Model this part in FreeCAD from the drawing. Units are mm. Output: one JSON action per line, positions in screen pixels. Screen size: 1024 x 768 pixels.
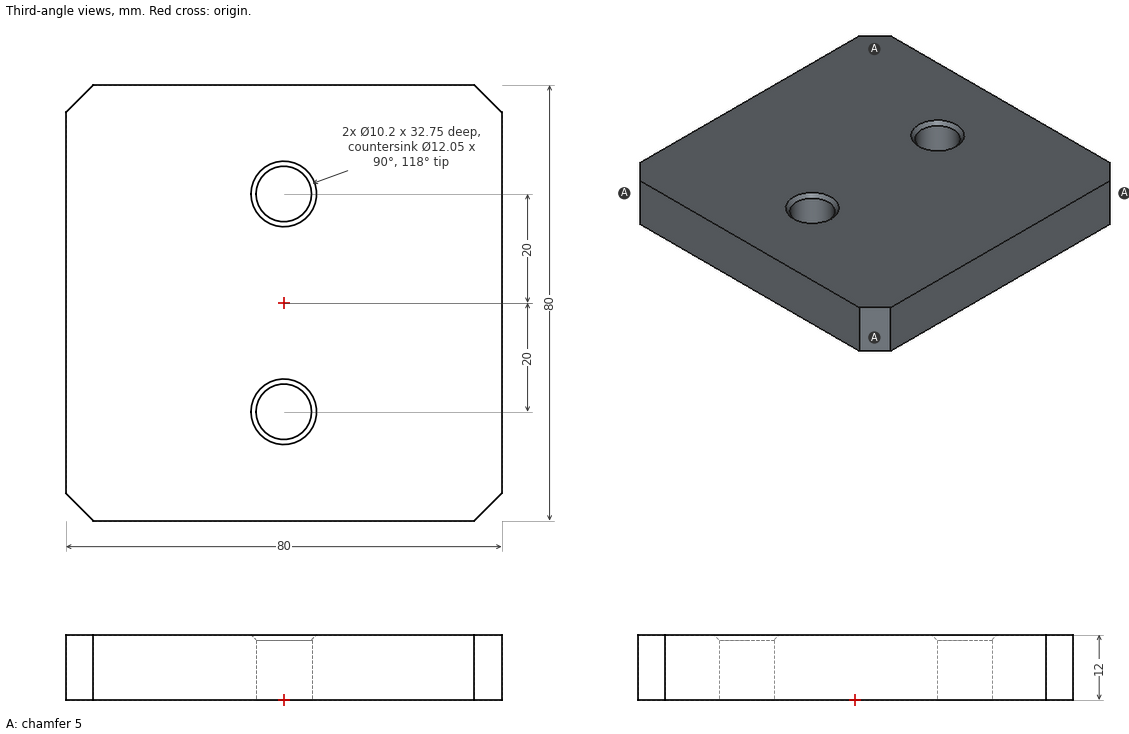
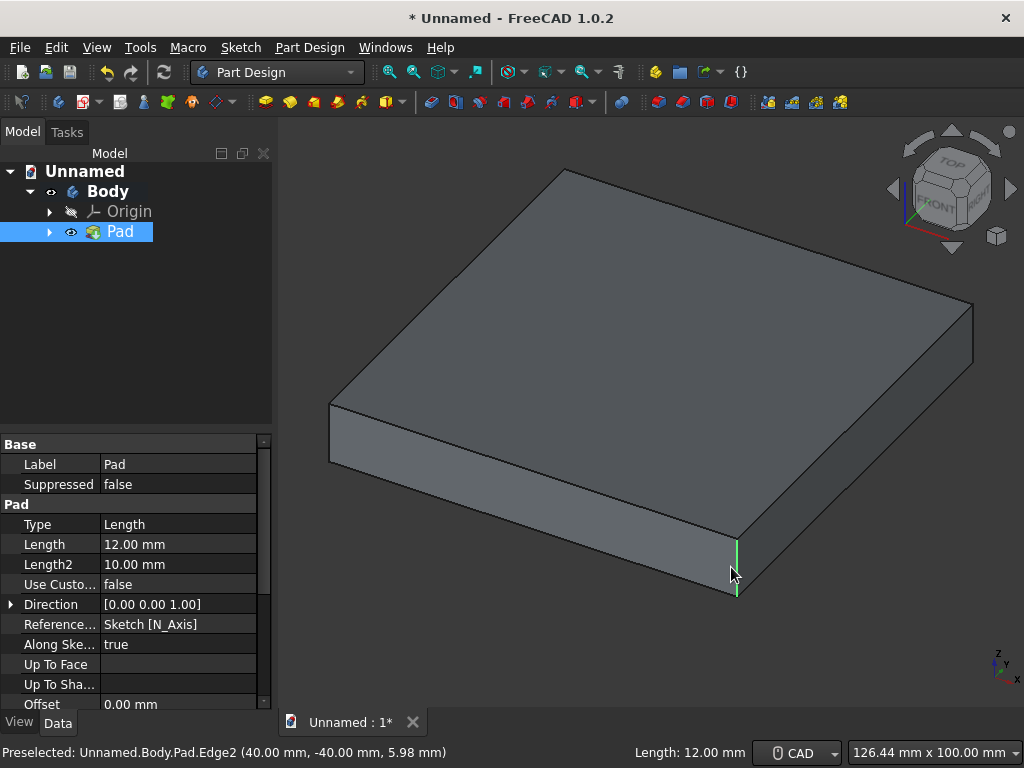
{"action": "key", "text": "0"}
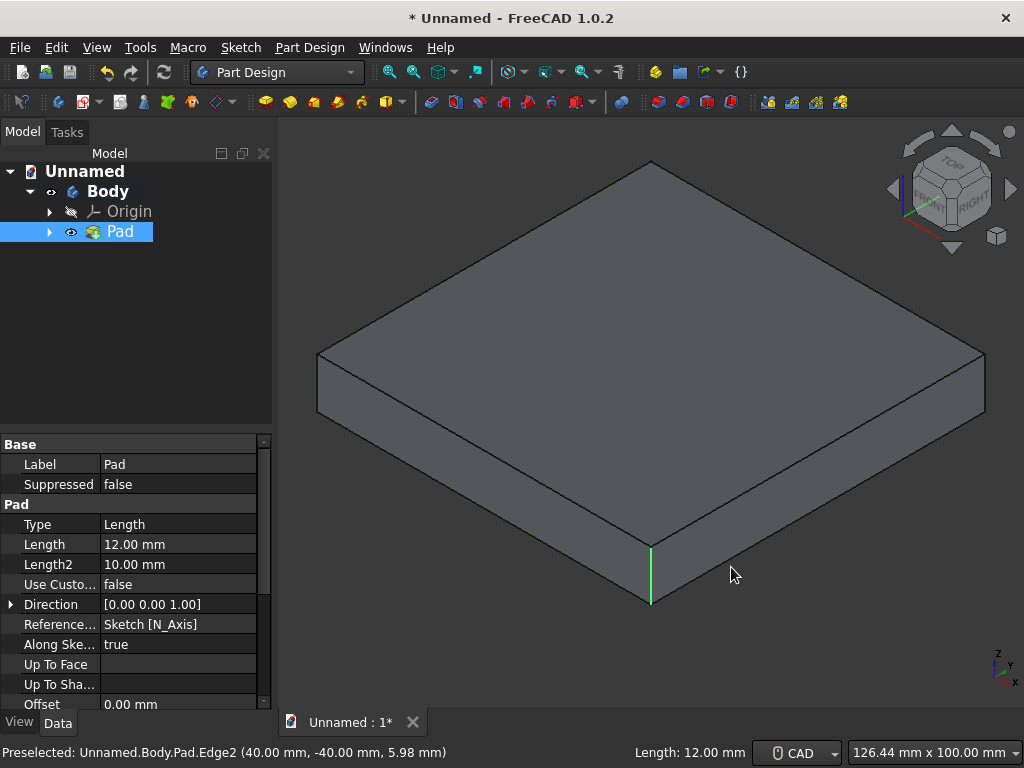
{"action": "key", "text": "2"}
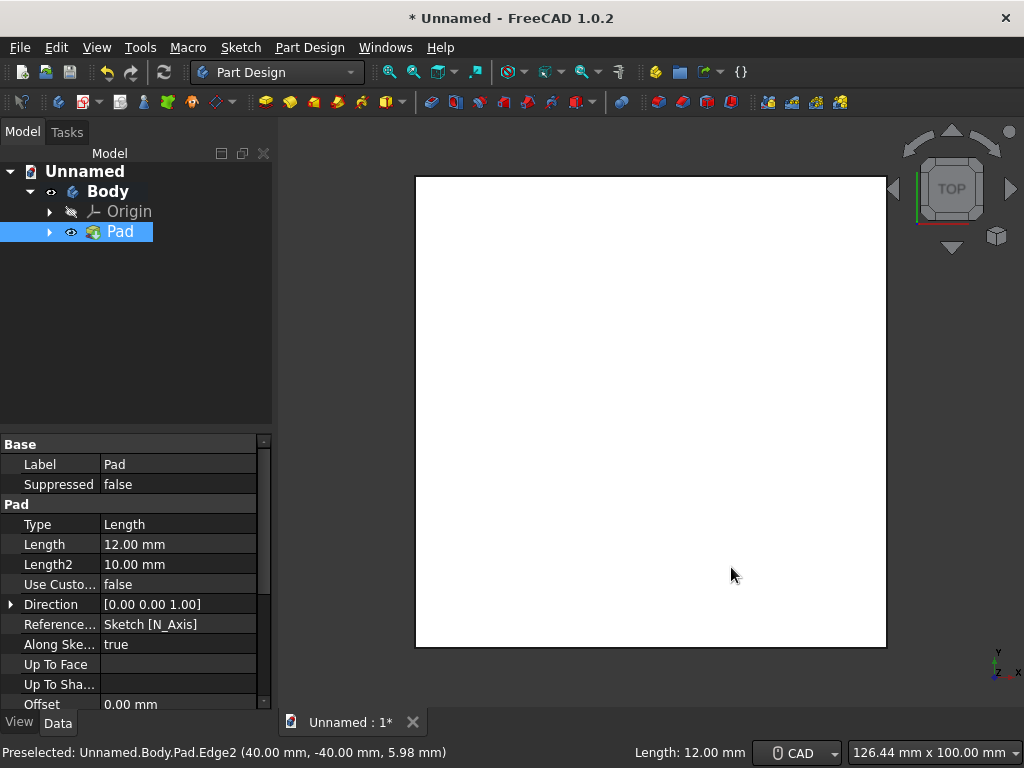
{"action": "key", "text": "1"}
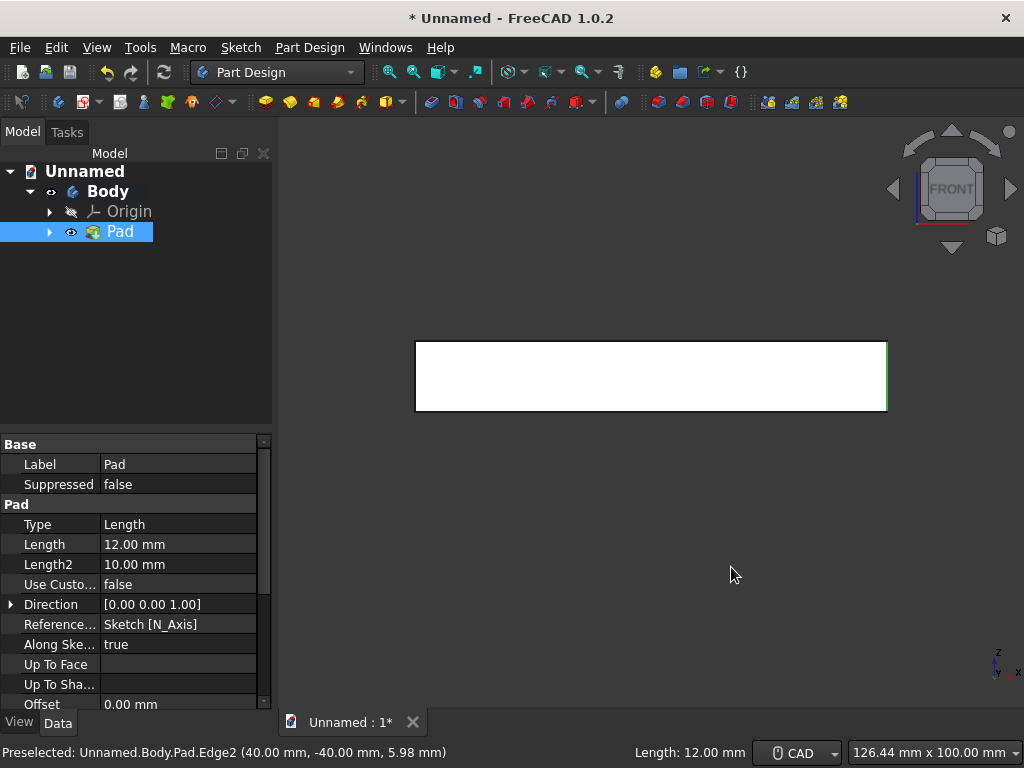
{"action": "left_click", "coordinate": [415, 376], "text": "ctrl"}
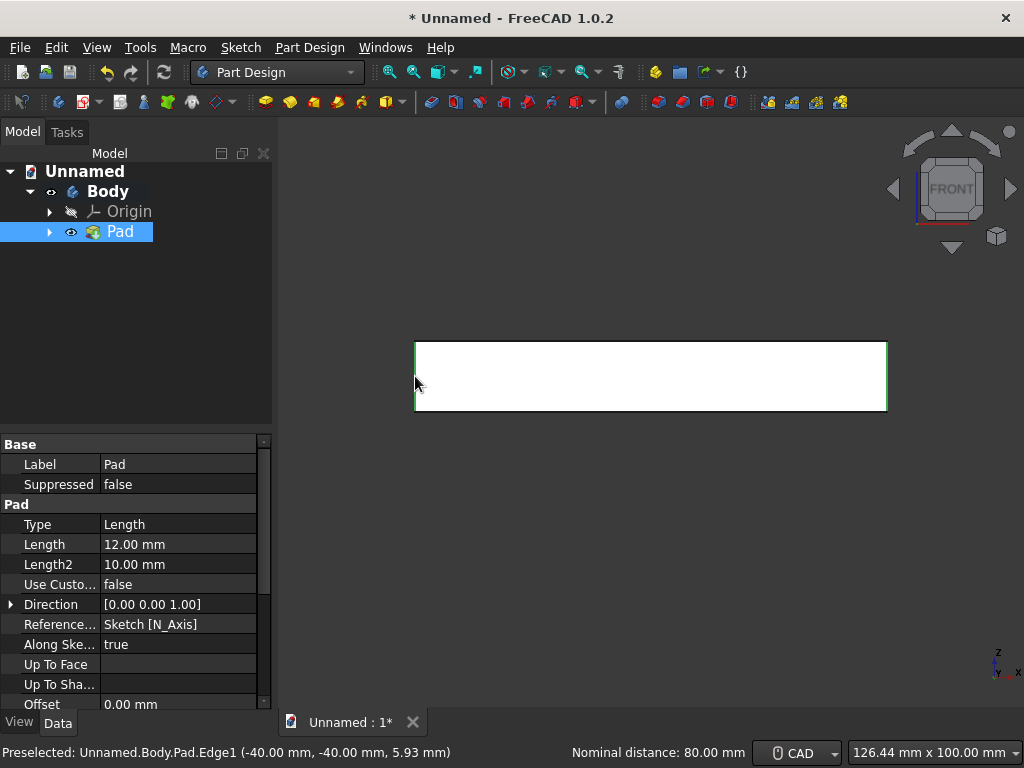
{"action": "key", "text": "3"}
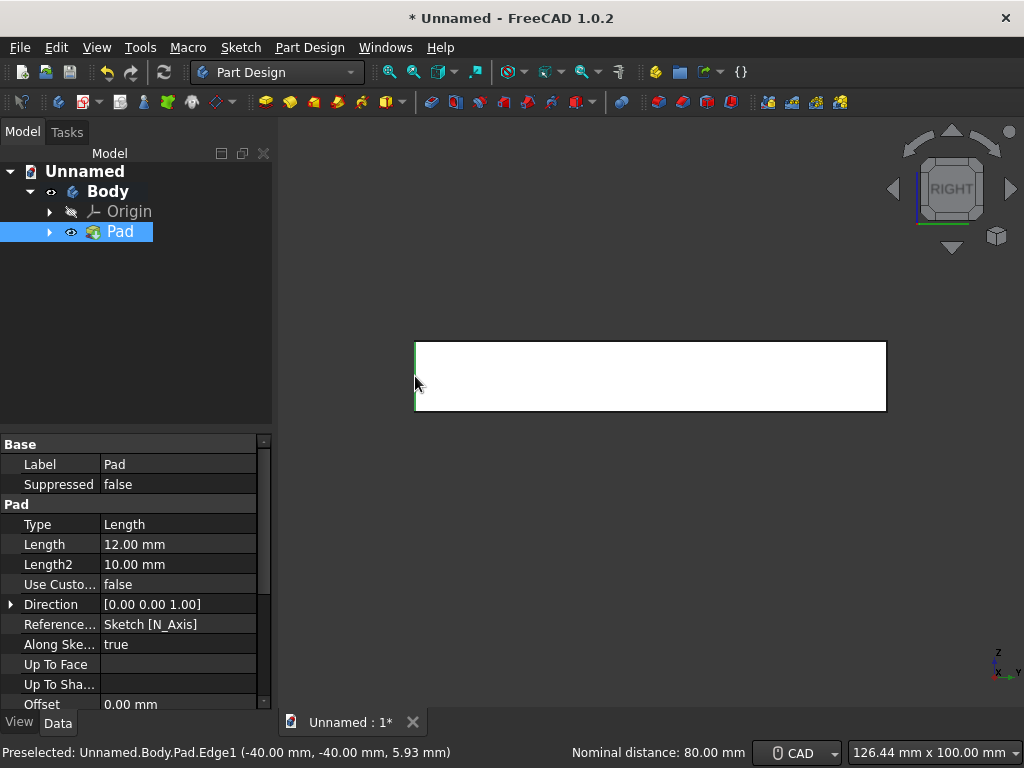
{"action": "left_click", "coordinate": [887, 376], "text": "ctrl"}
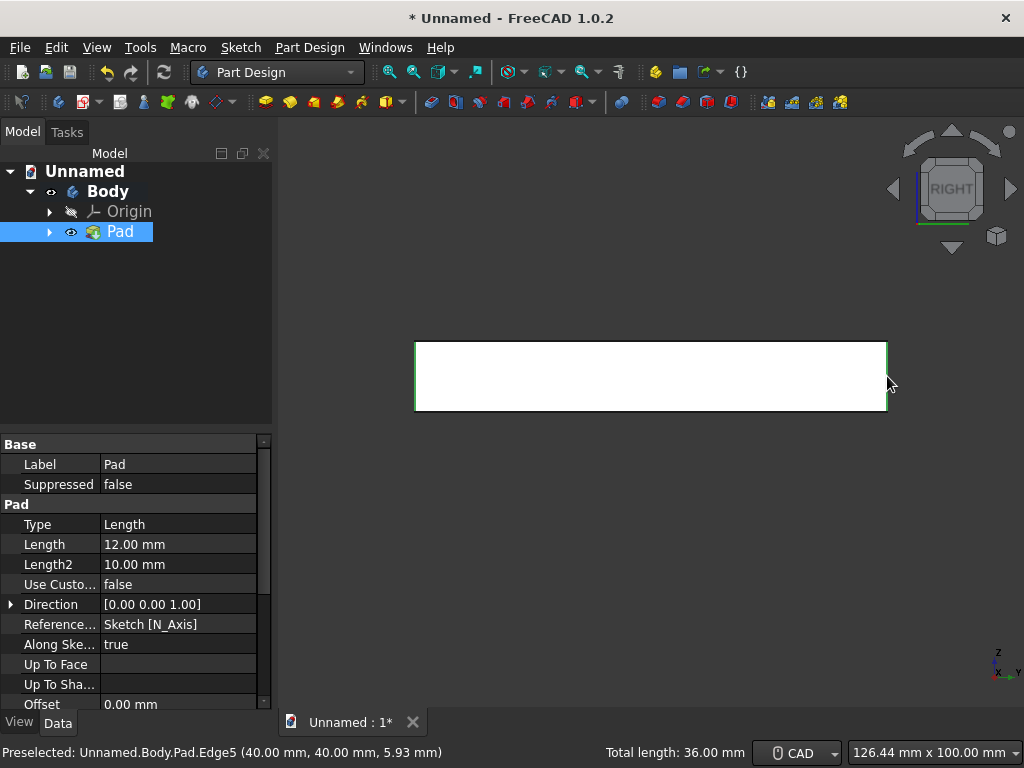
{"action": "key", "text": "5"}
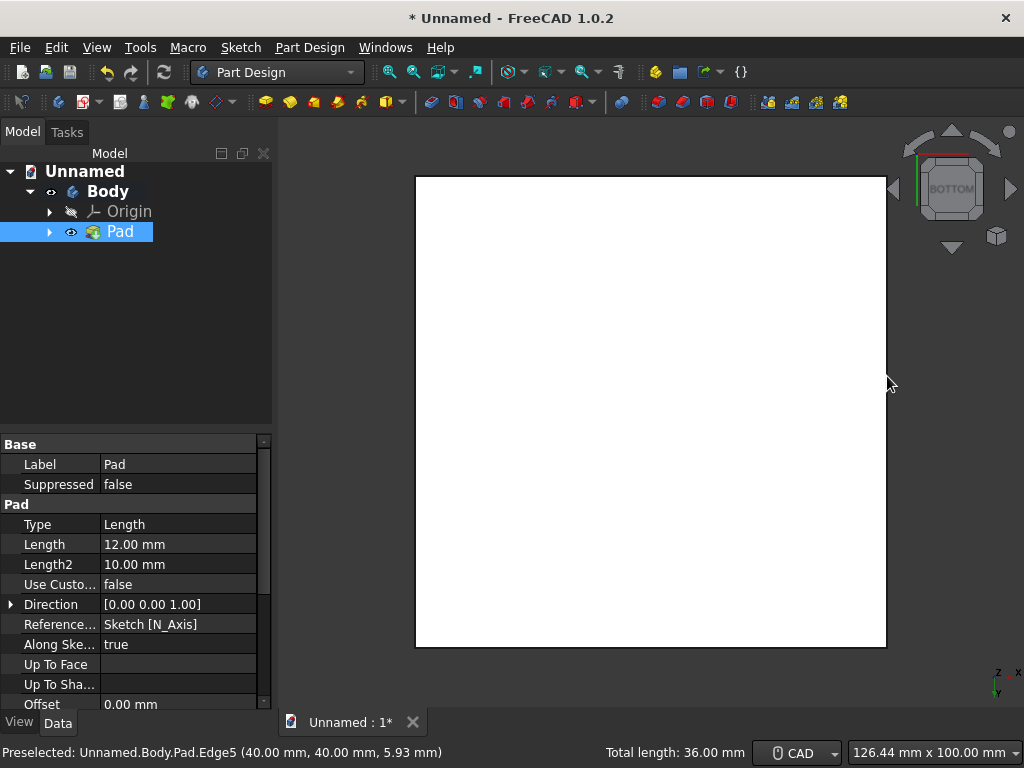
{"action": "key", "text": "4"}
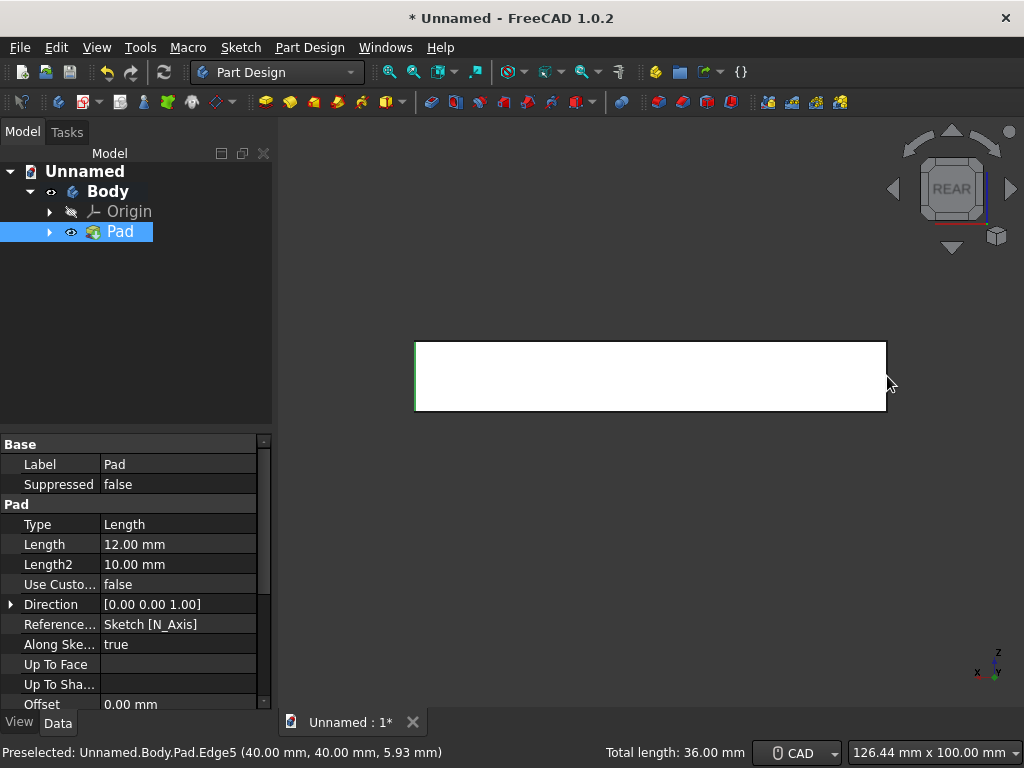
{"action": "left_click", "coordinate": [887, 376], "text": "ctrl"}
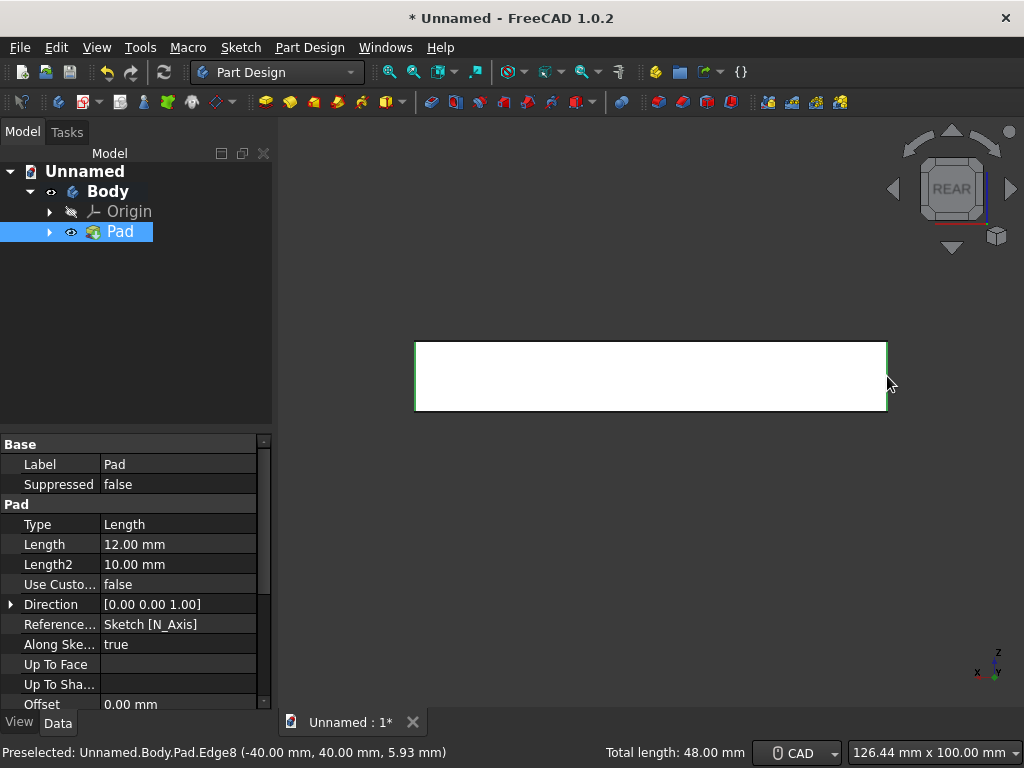
{"action": "left_click", "coordinate": [684, 102]}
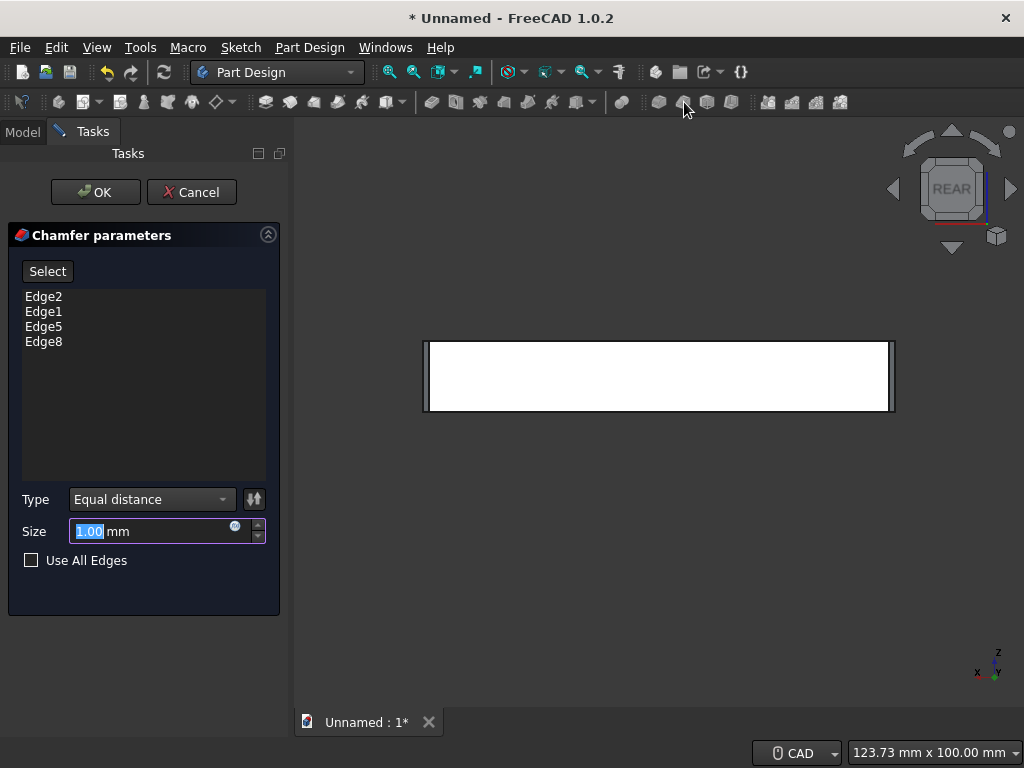
{"action": "type", "text": "5"}
{"action": "key", "text": "Tab"}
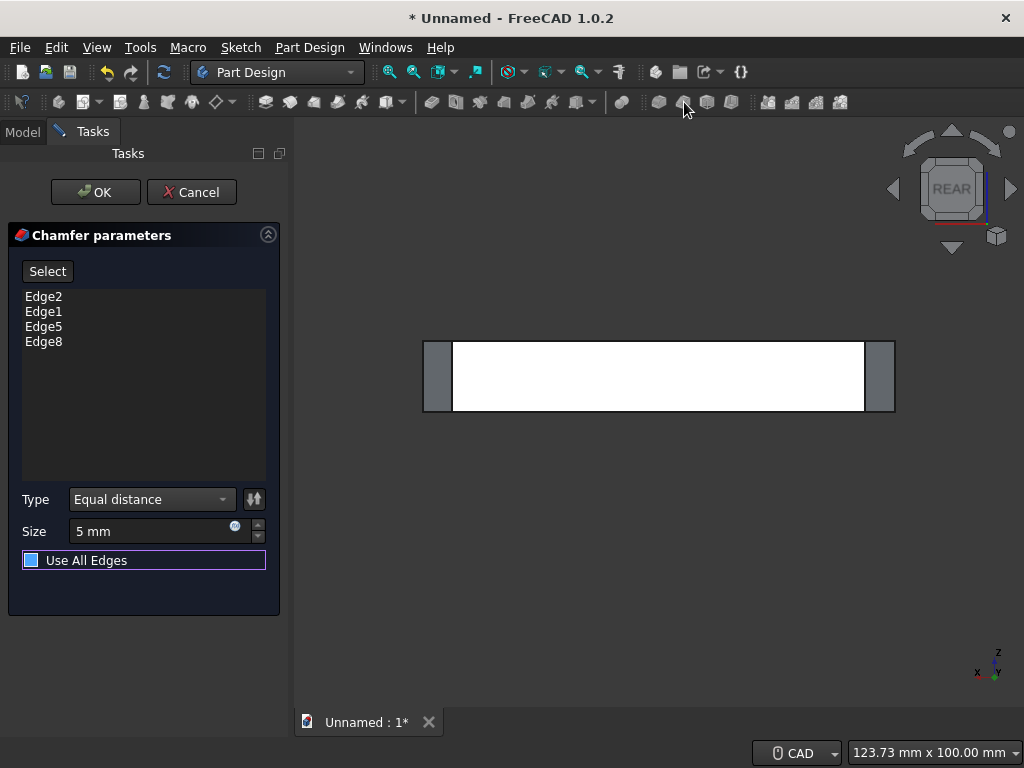
{"action": "left_click", "coordinate": [96, 192]}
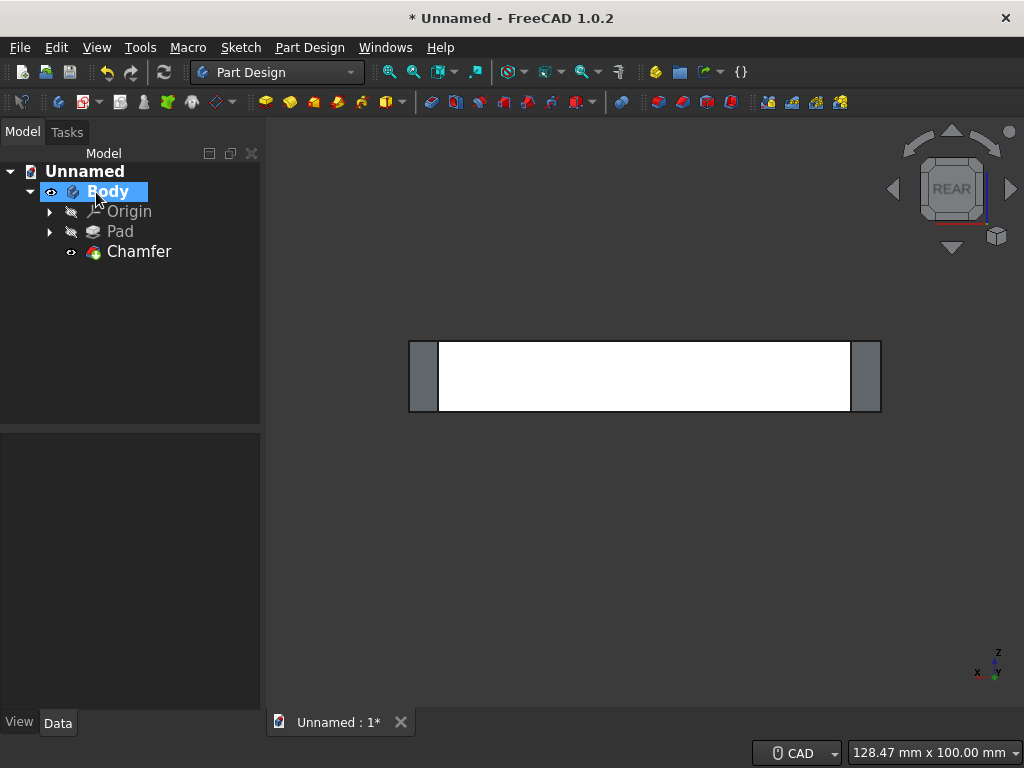
{"action": "key", "text": "0"}